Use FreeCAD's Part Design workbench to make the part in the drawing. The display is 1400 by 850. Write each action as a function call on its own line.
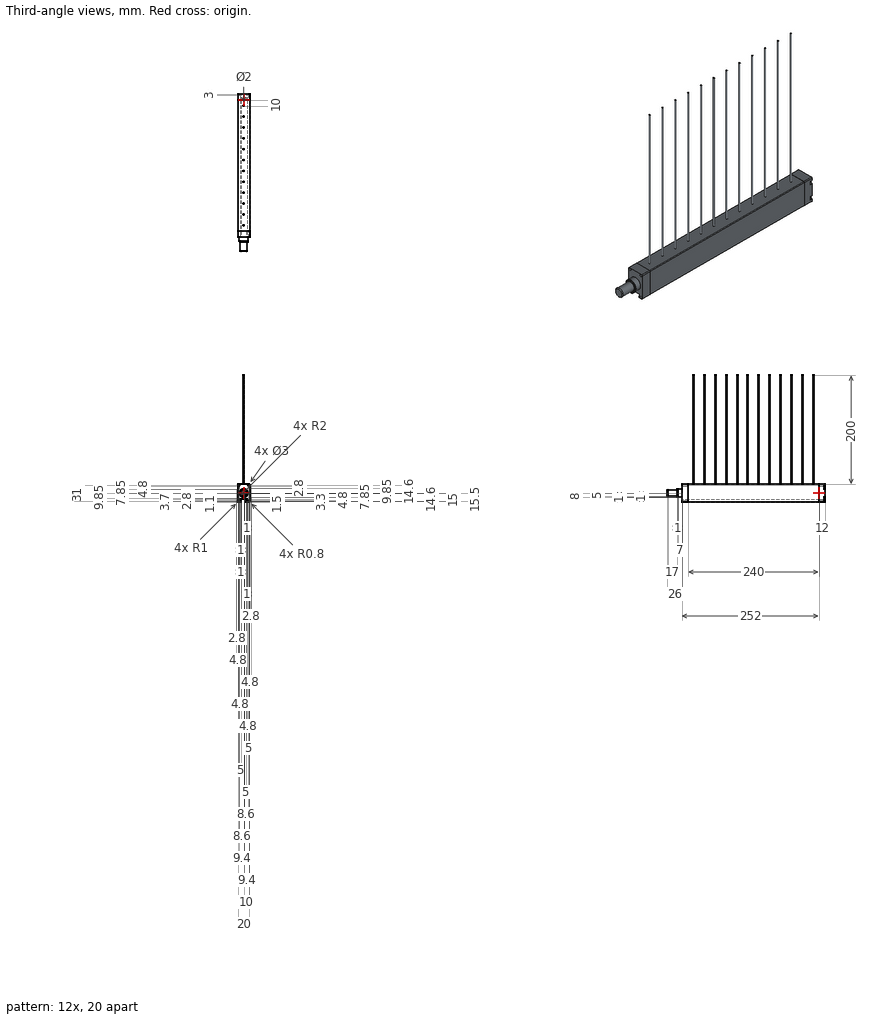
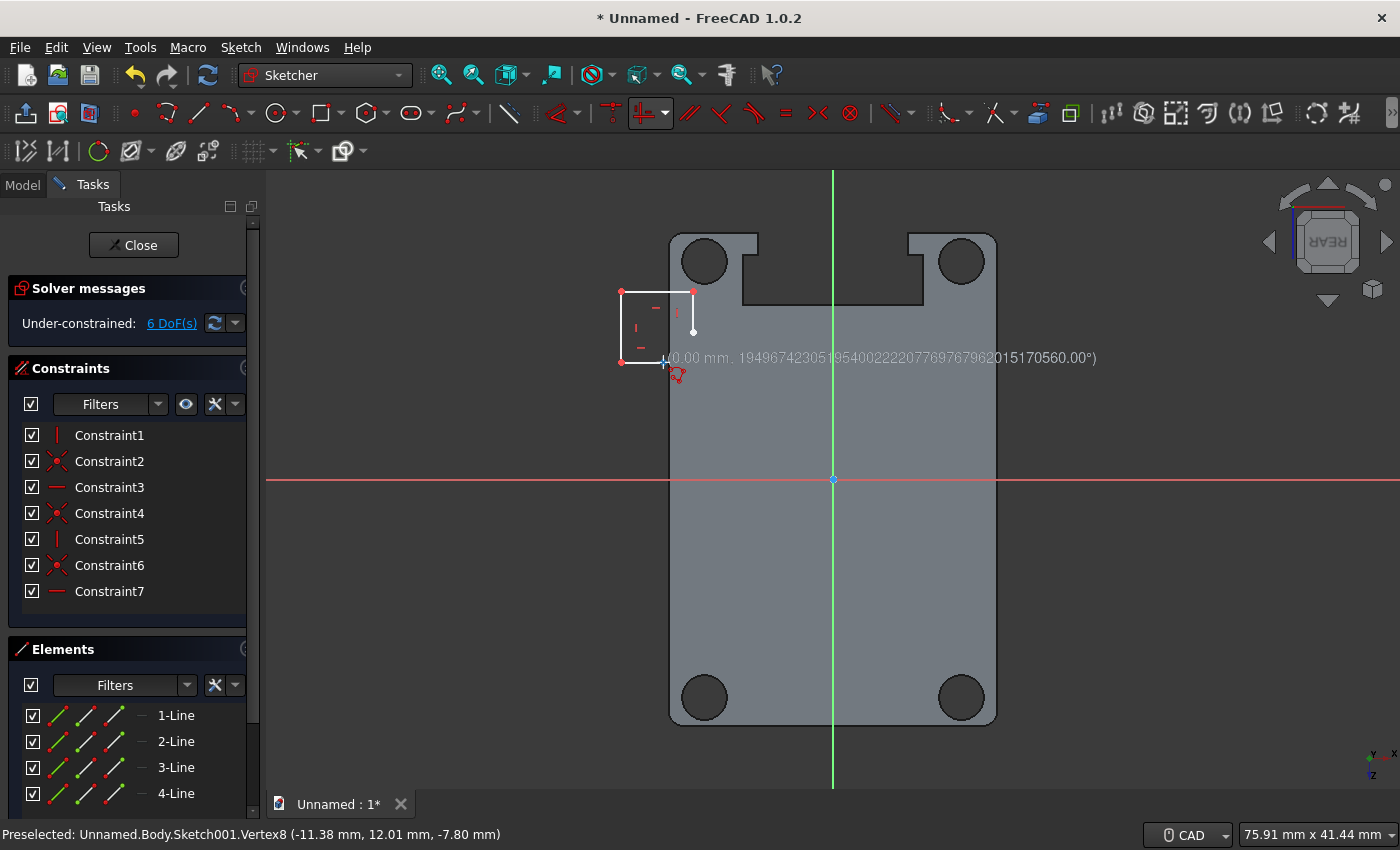
click(232, 114)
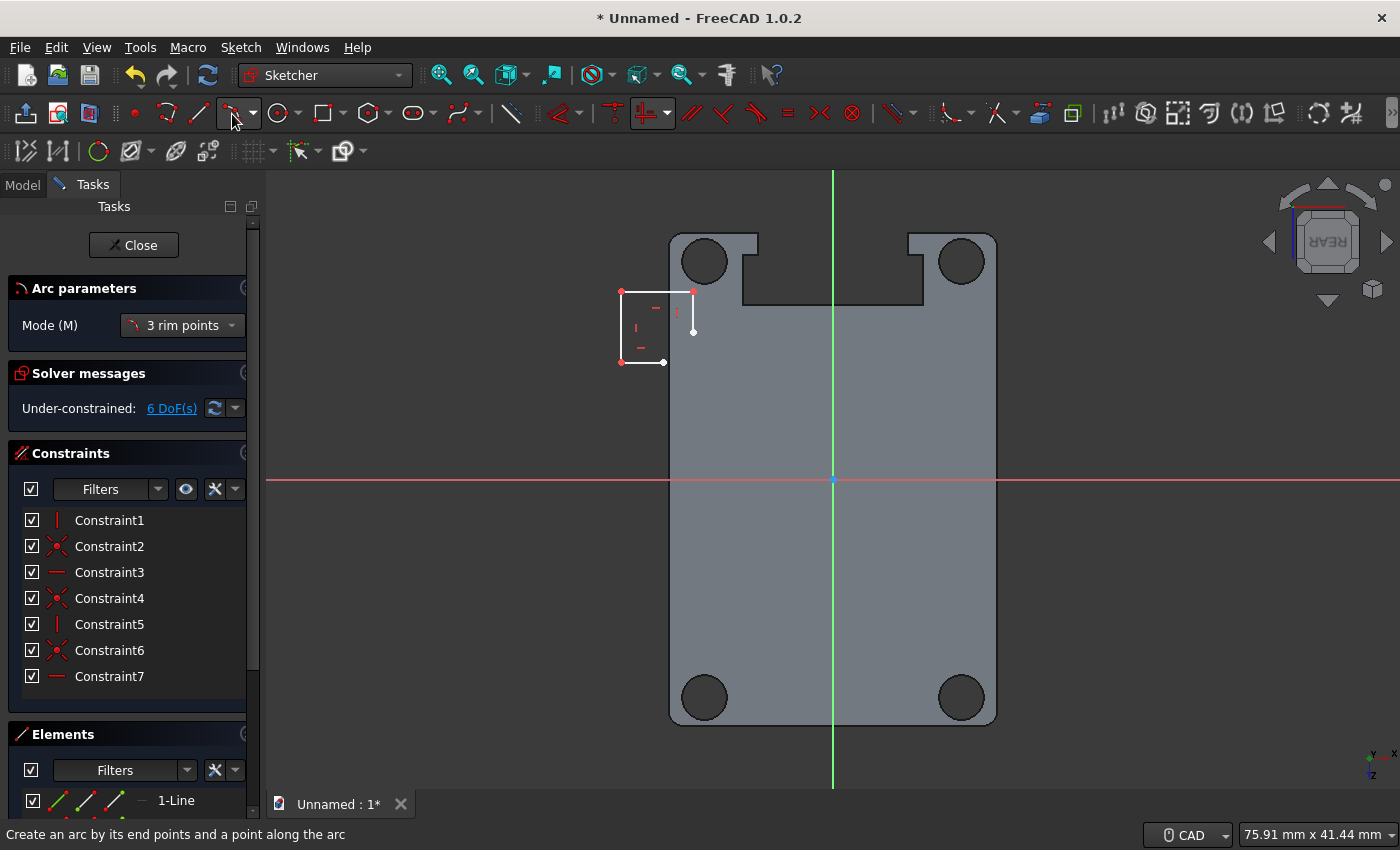
click(663, 363)
click(693, 333)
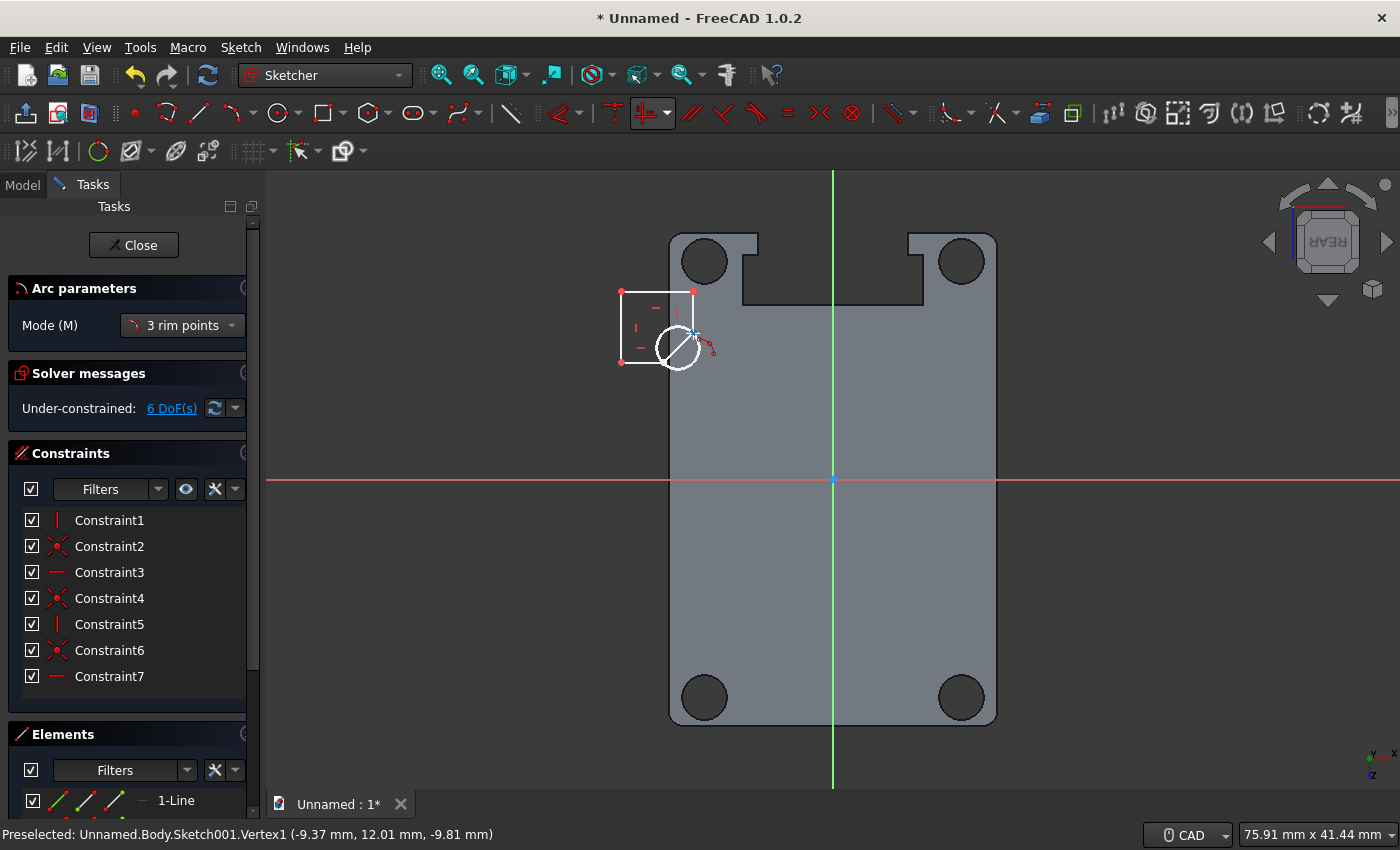
scroll(684, 353, up, 3)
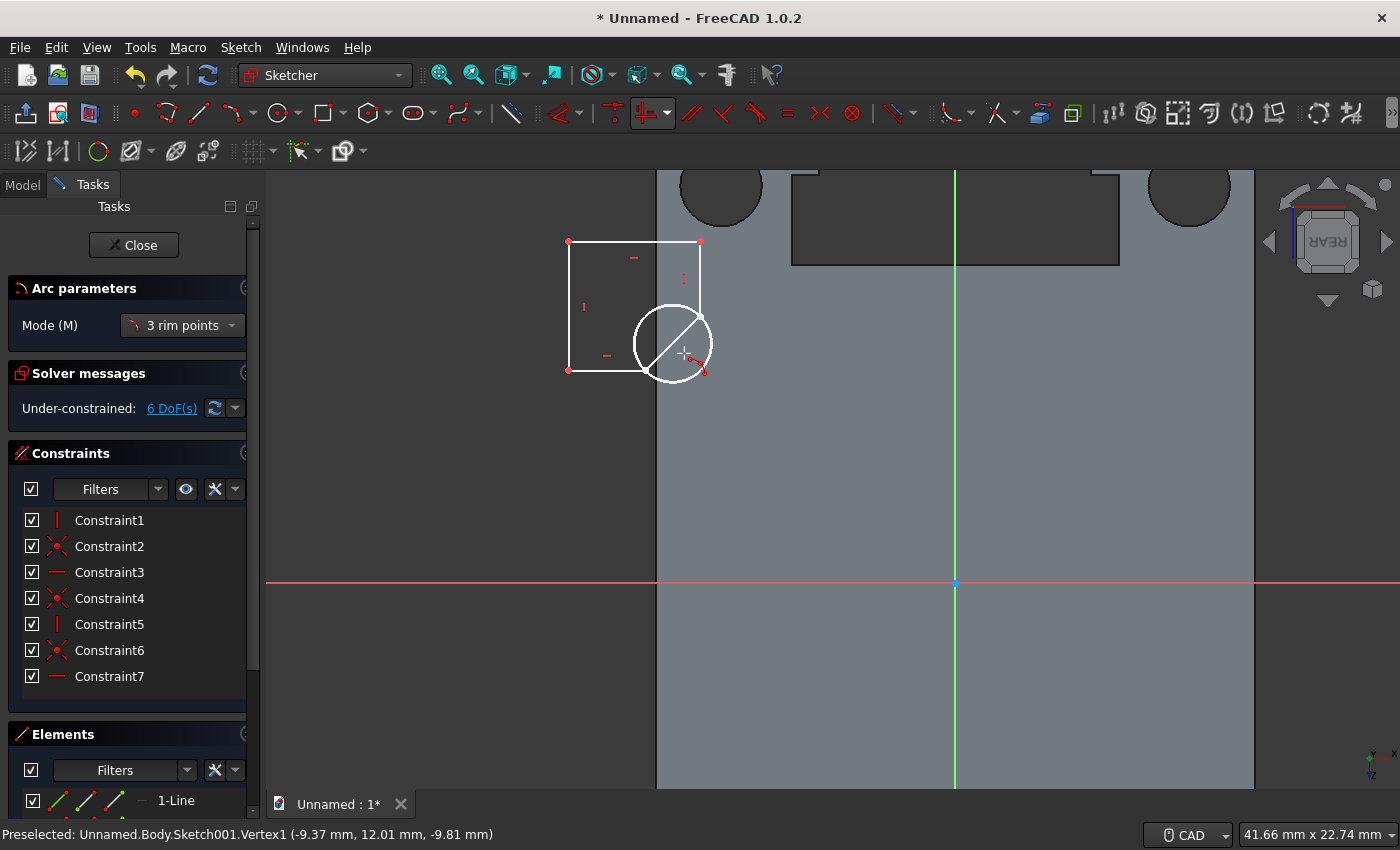
click(683, 354)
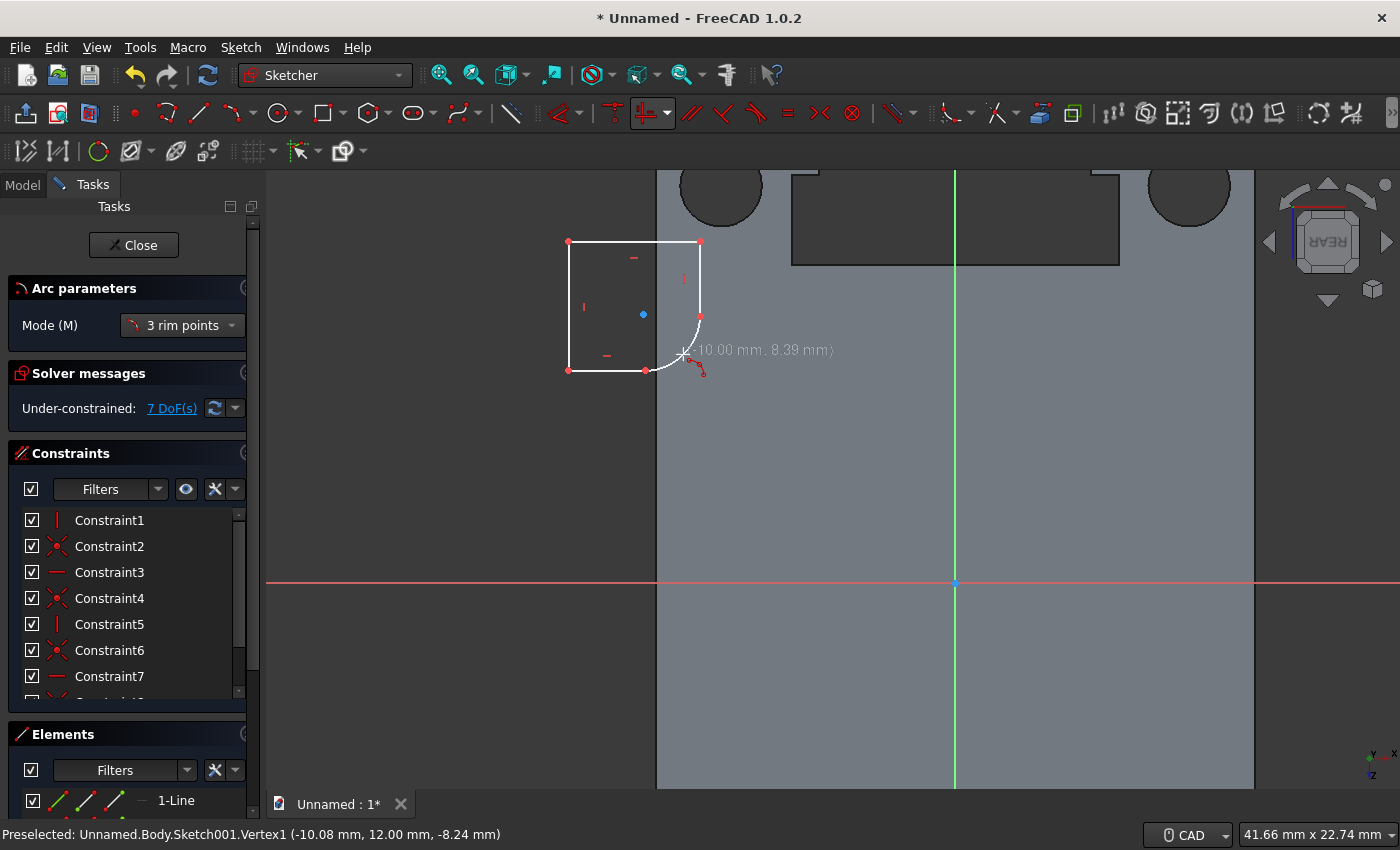
click(168, 114)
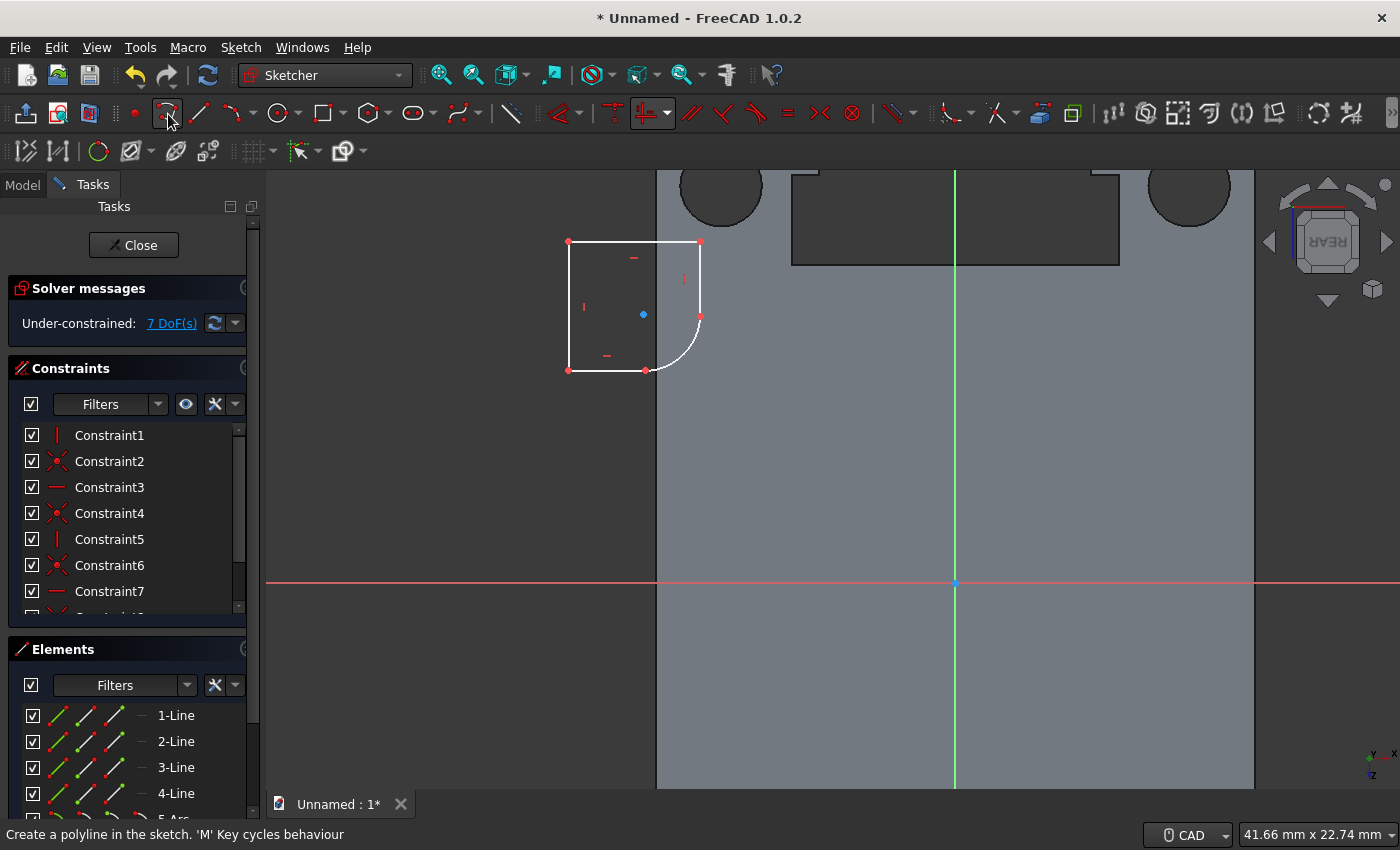
scroll(533, 353, down, 3)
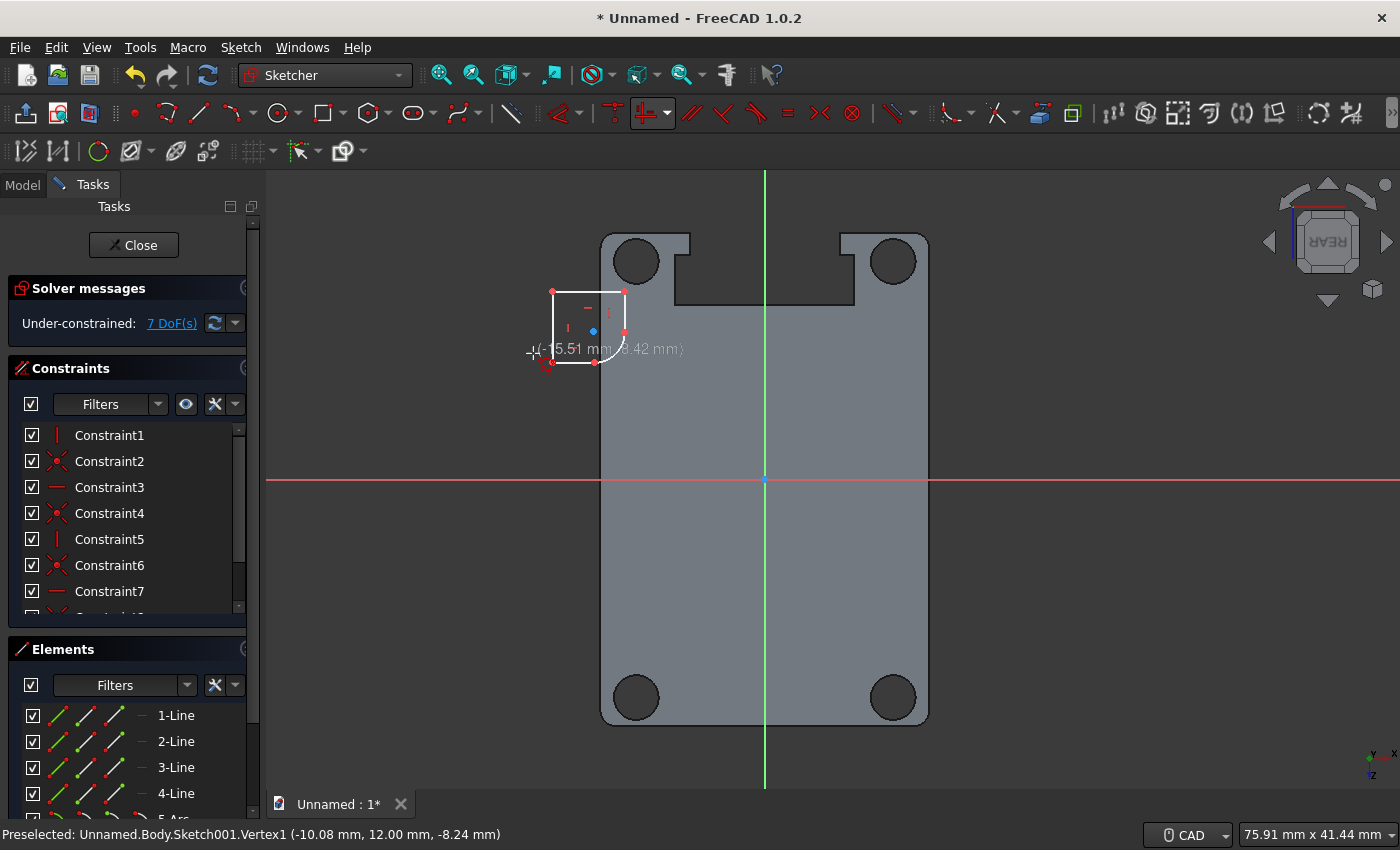
click(935, 362)
click(977, 362)
click(977, 291)
click(905, 291)
click(905, 332)
right_click(905, 332)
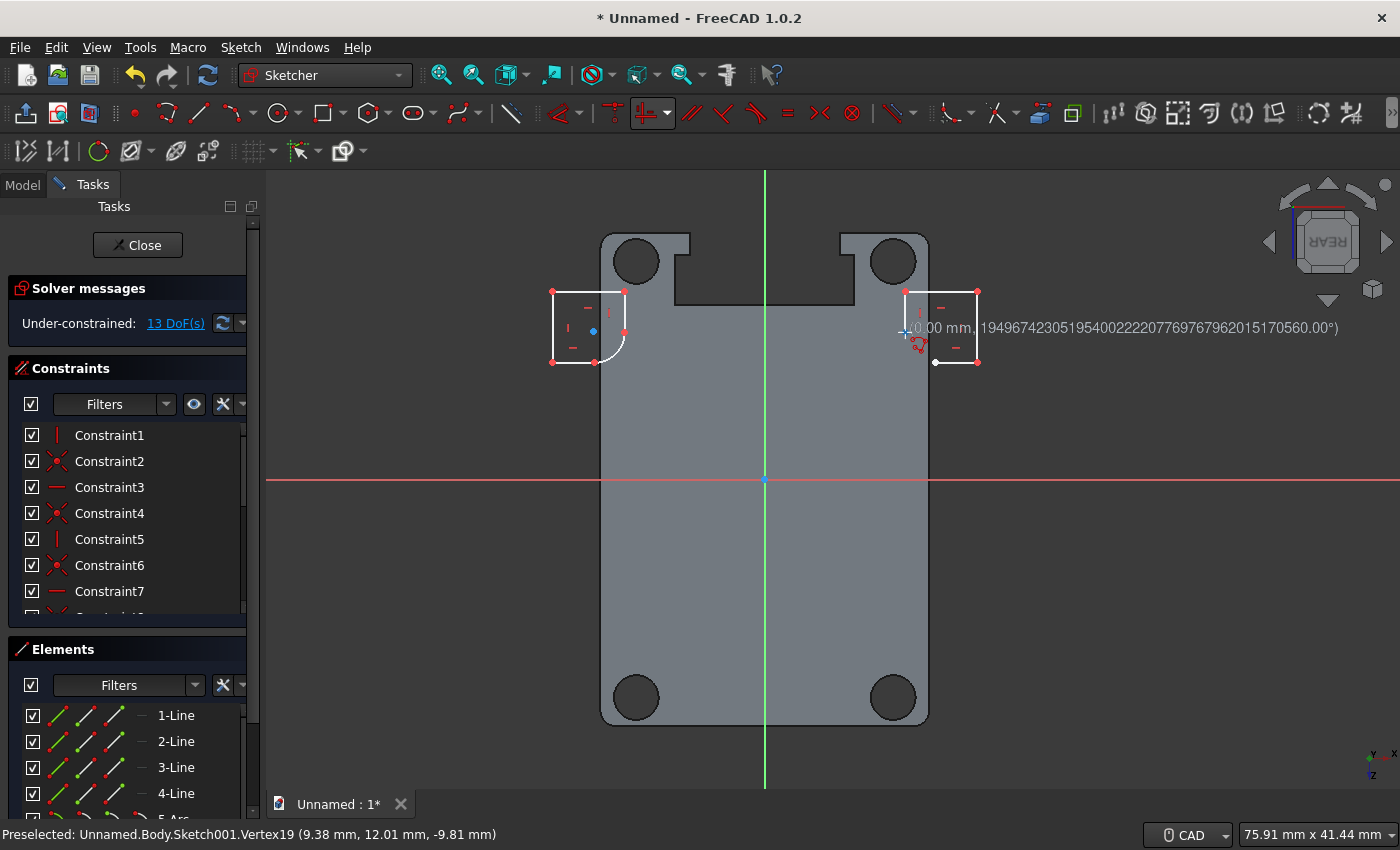
key(g)
key(3)
key(a)